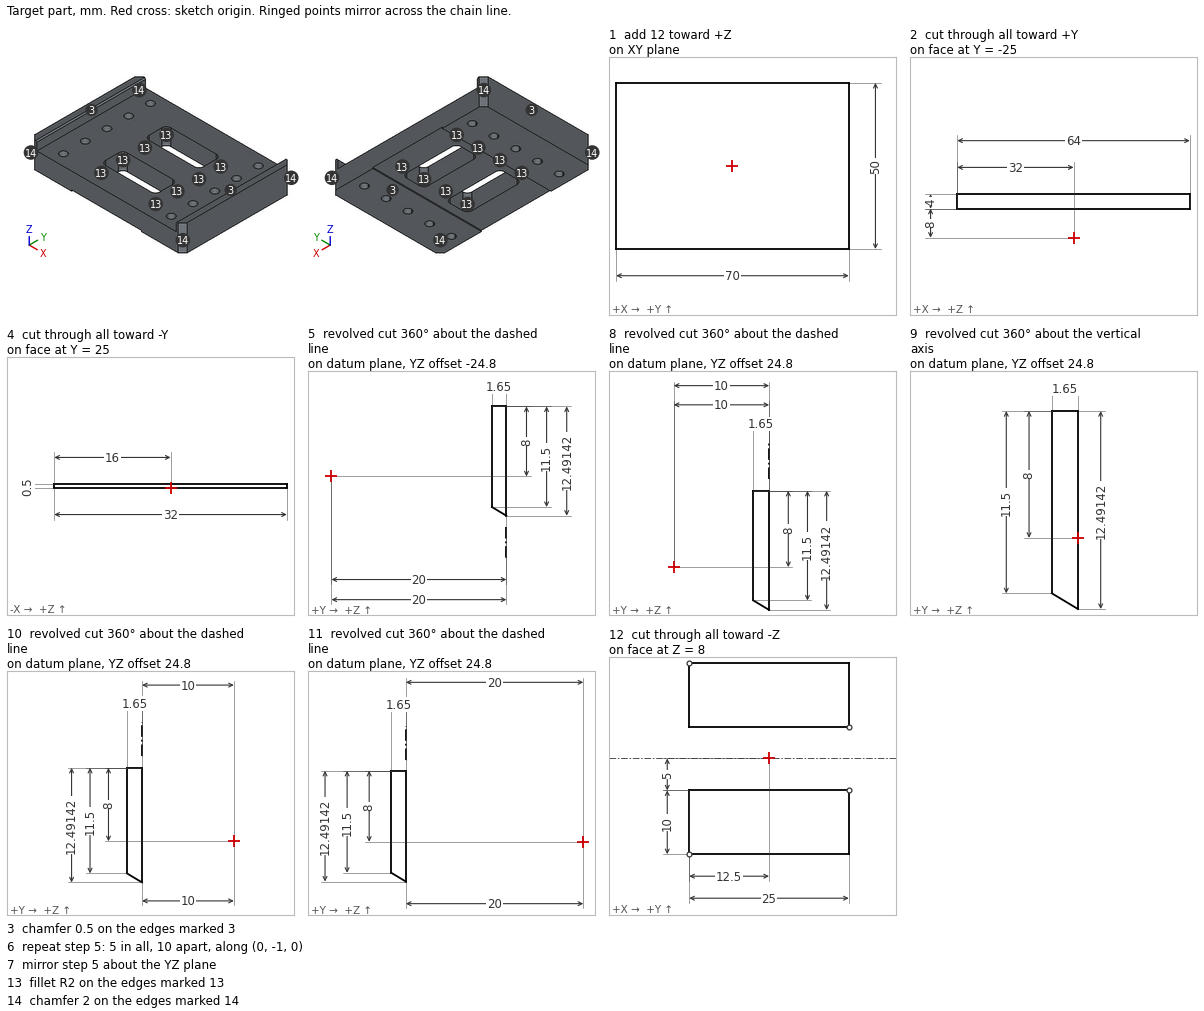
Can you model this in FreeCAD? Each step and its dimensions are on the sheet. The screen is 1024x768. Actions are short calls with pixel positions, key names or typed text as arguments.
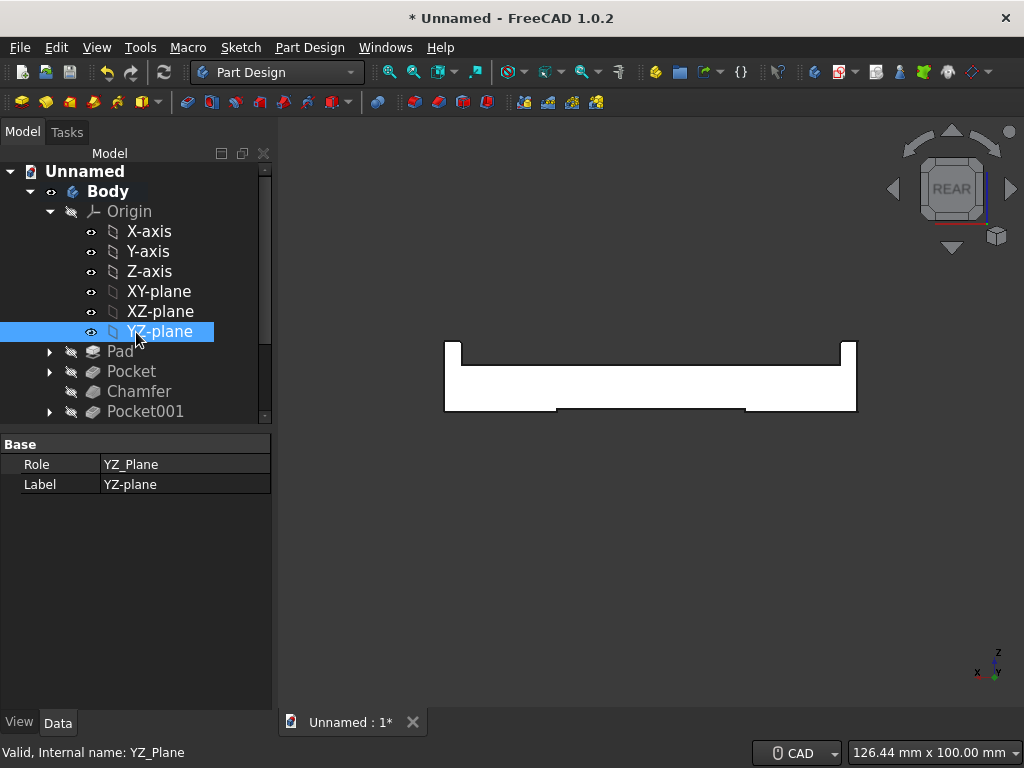
click(972, 72)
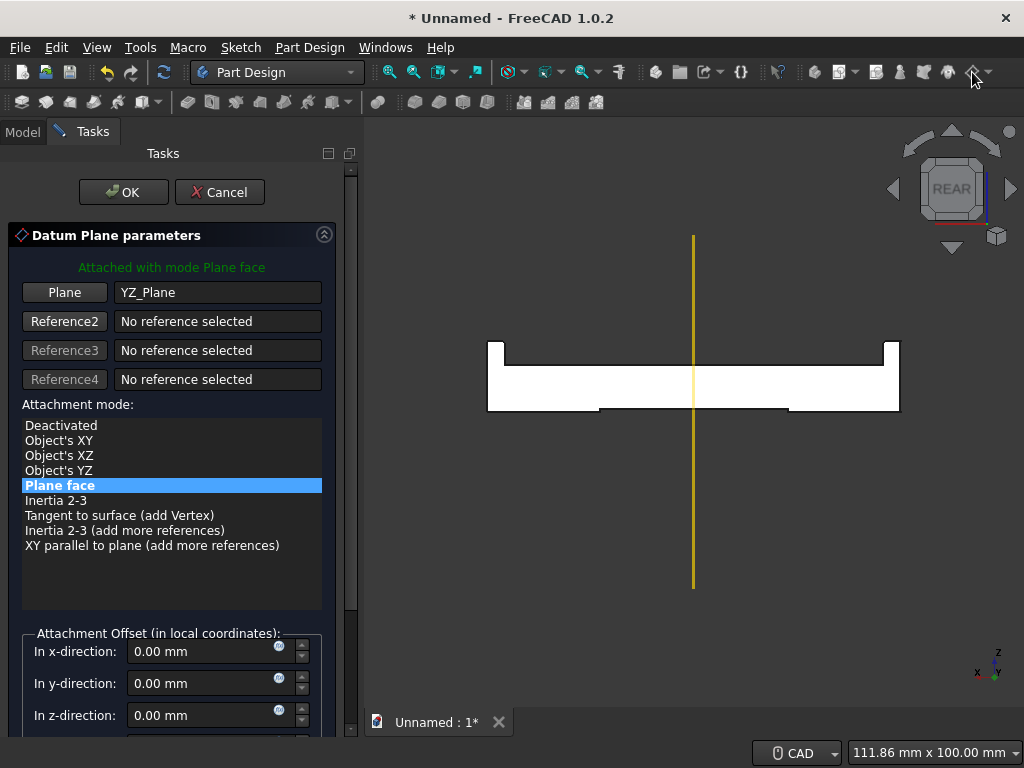
triple_click(210, 715)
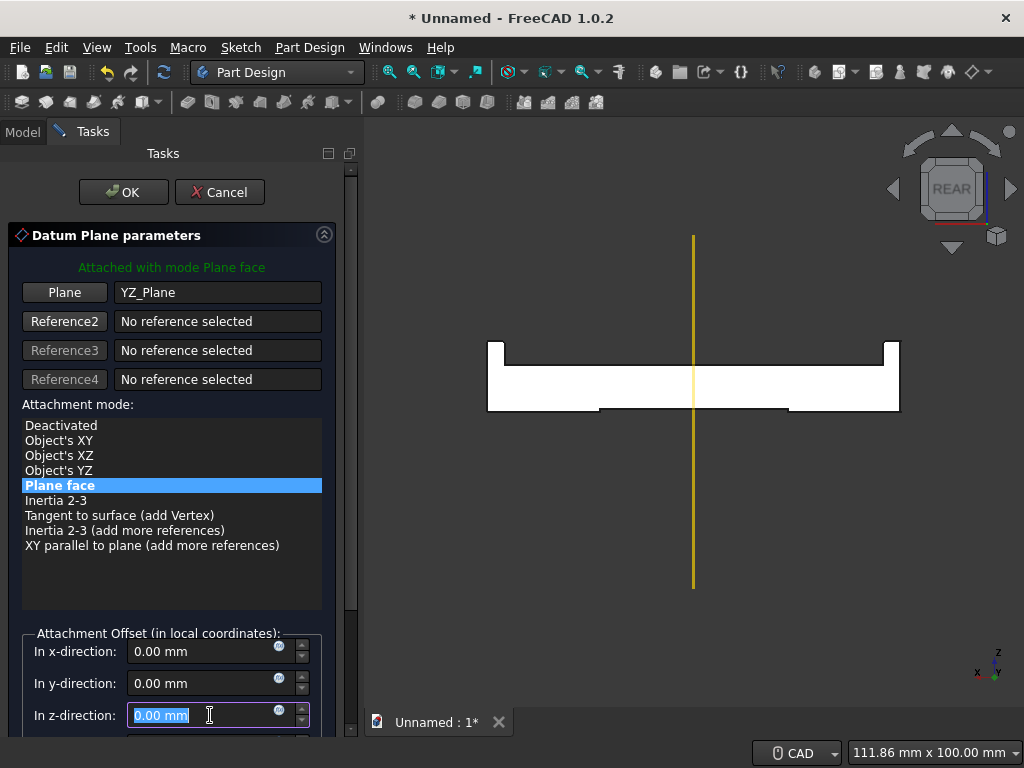
text(24.8)
key(Tab)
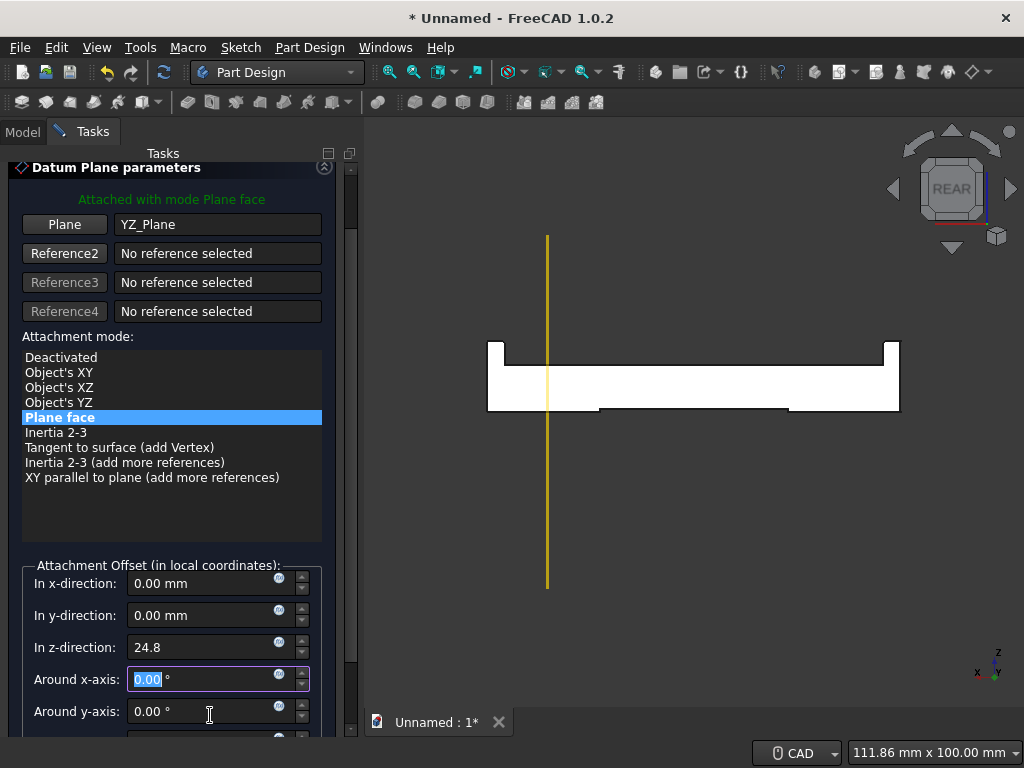
scroll(351, 450, up, 2)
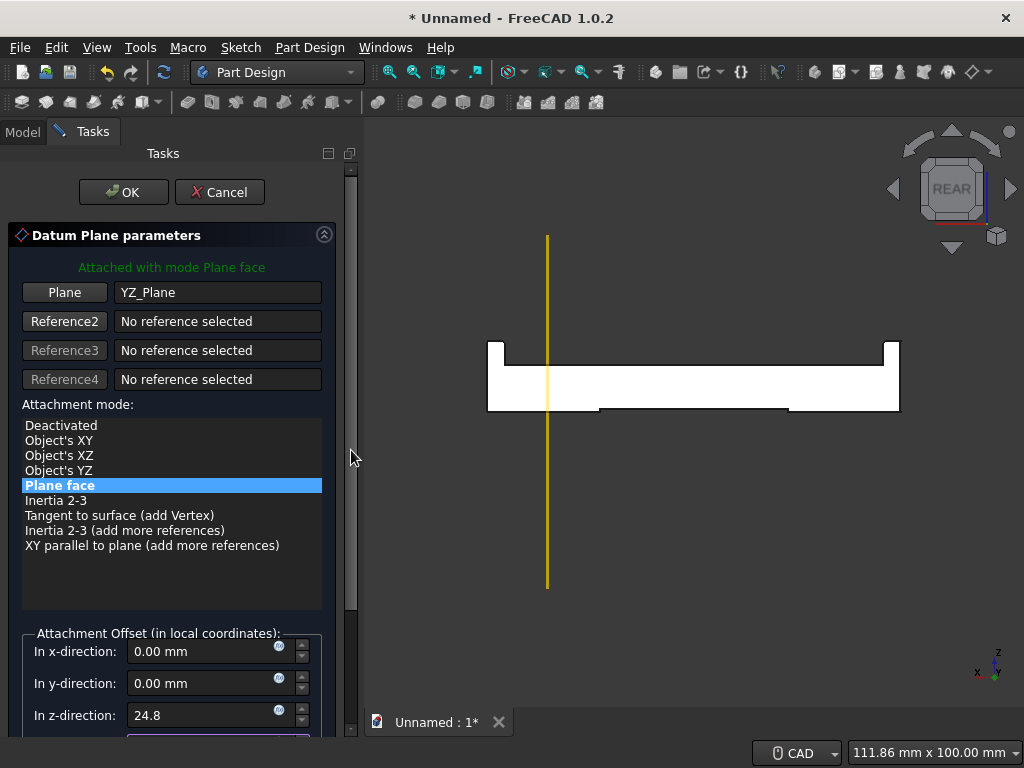
click(124, 192)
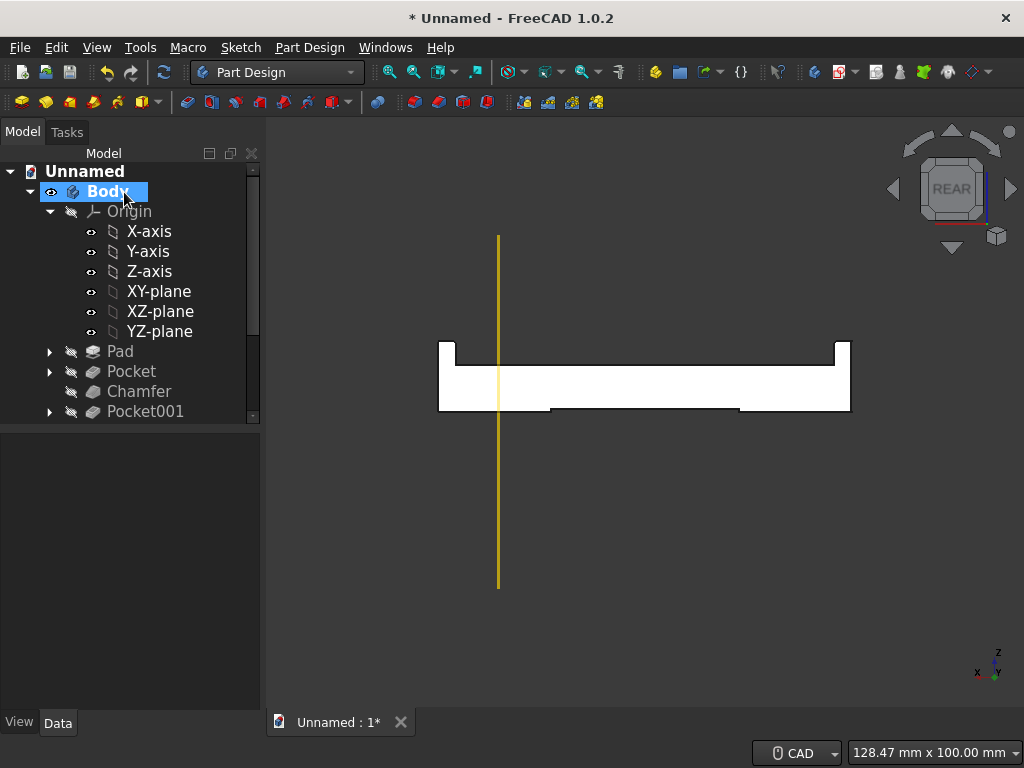
scroll(100, 287, down, 3)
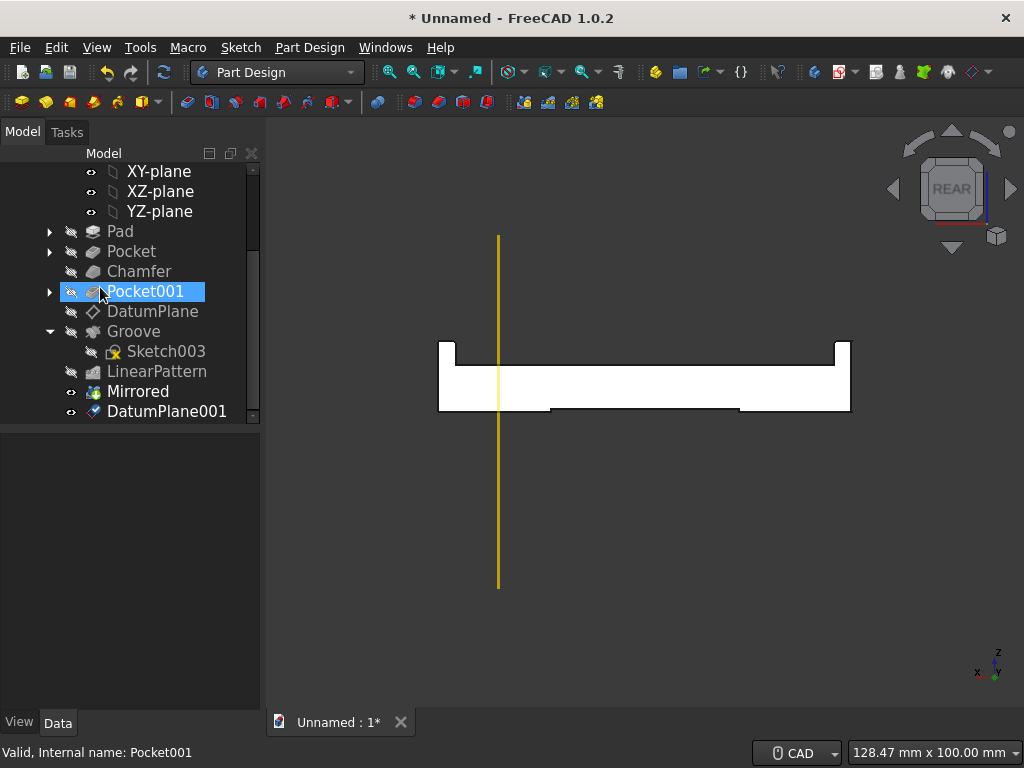
click(116, 412)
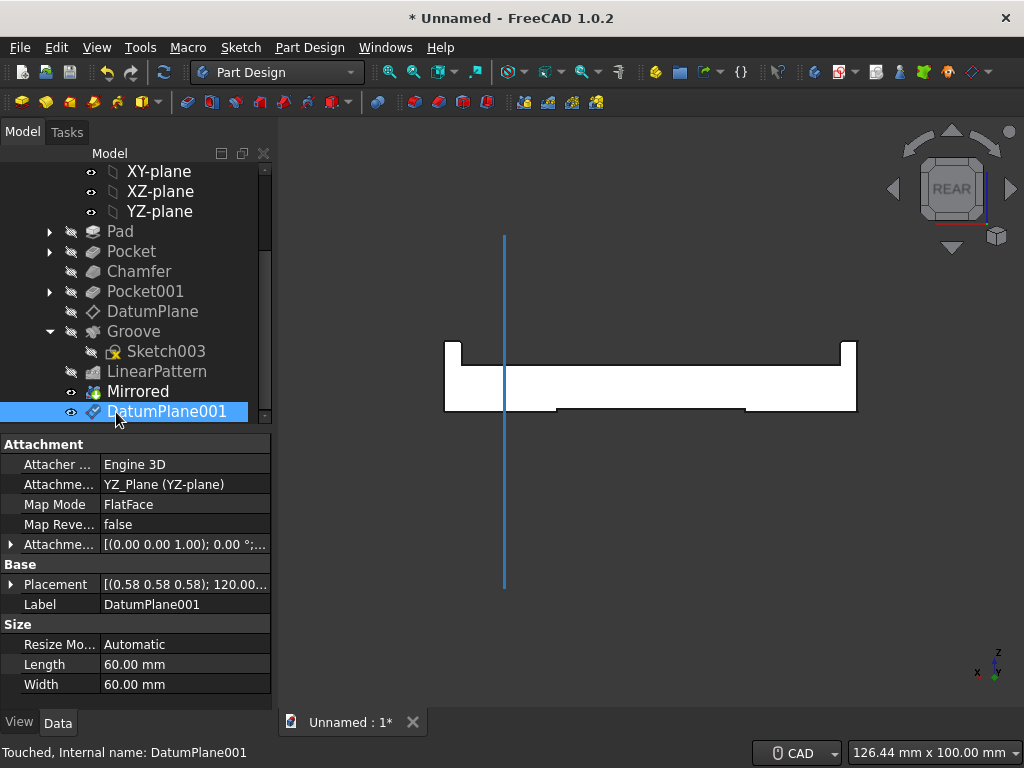
click(840, 72)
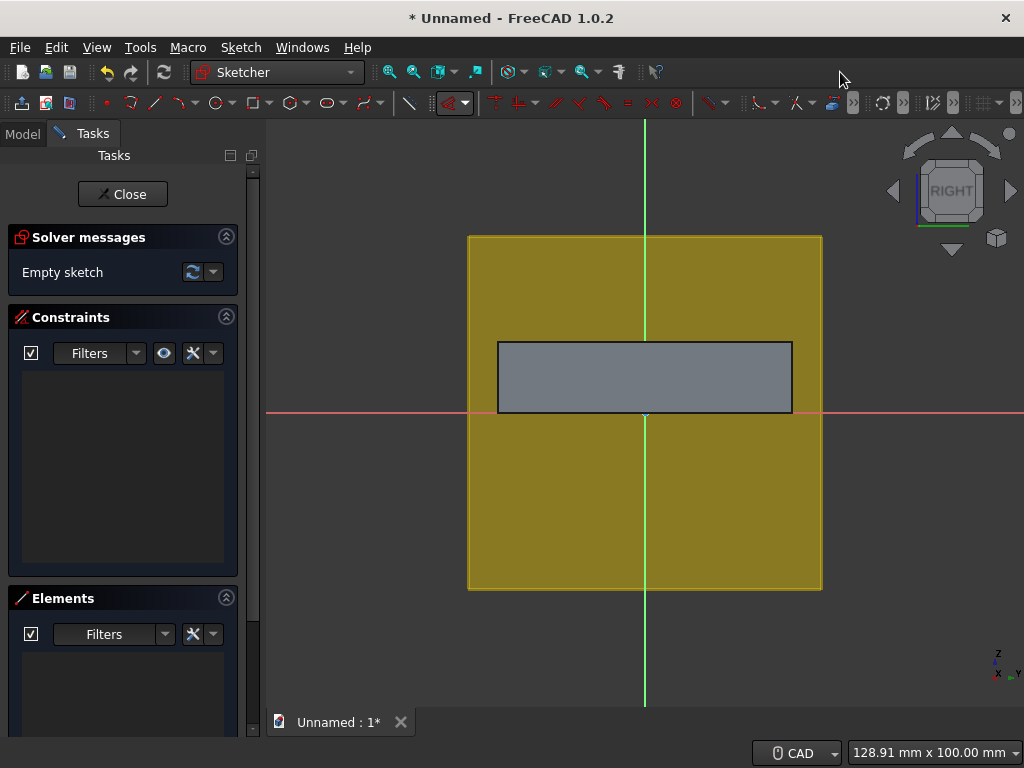
click(70, 104)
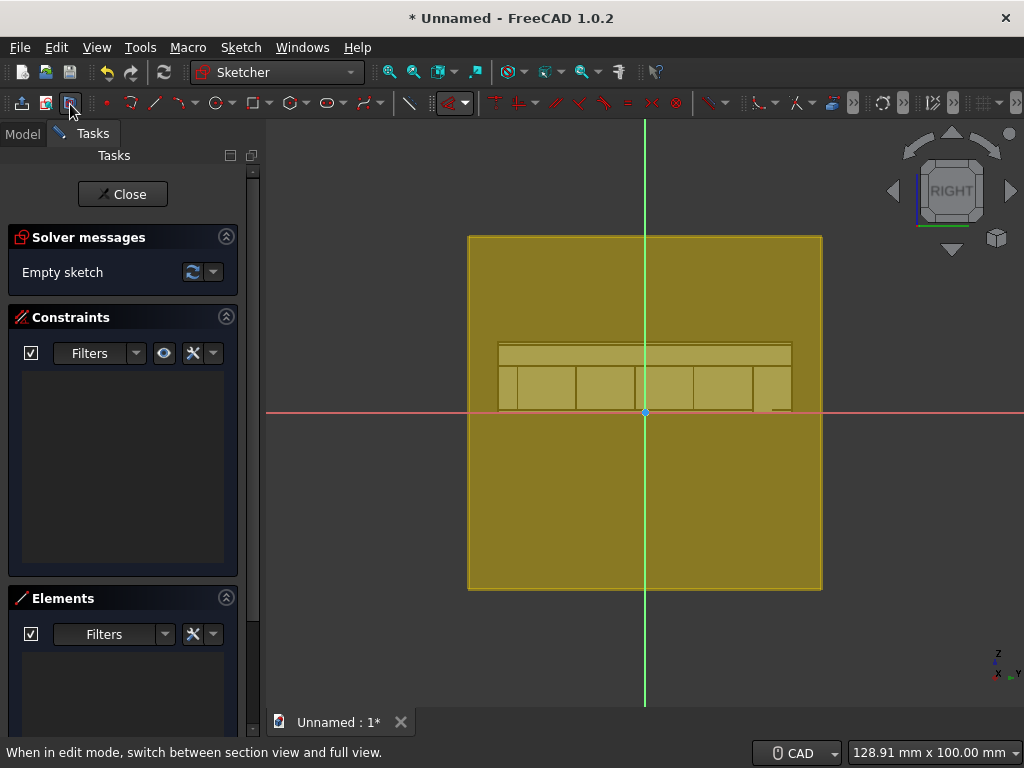
scroll(717, 377, up, 6)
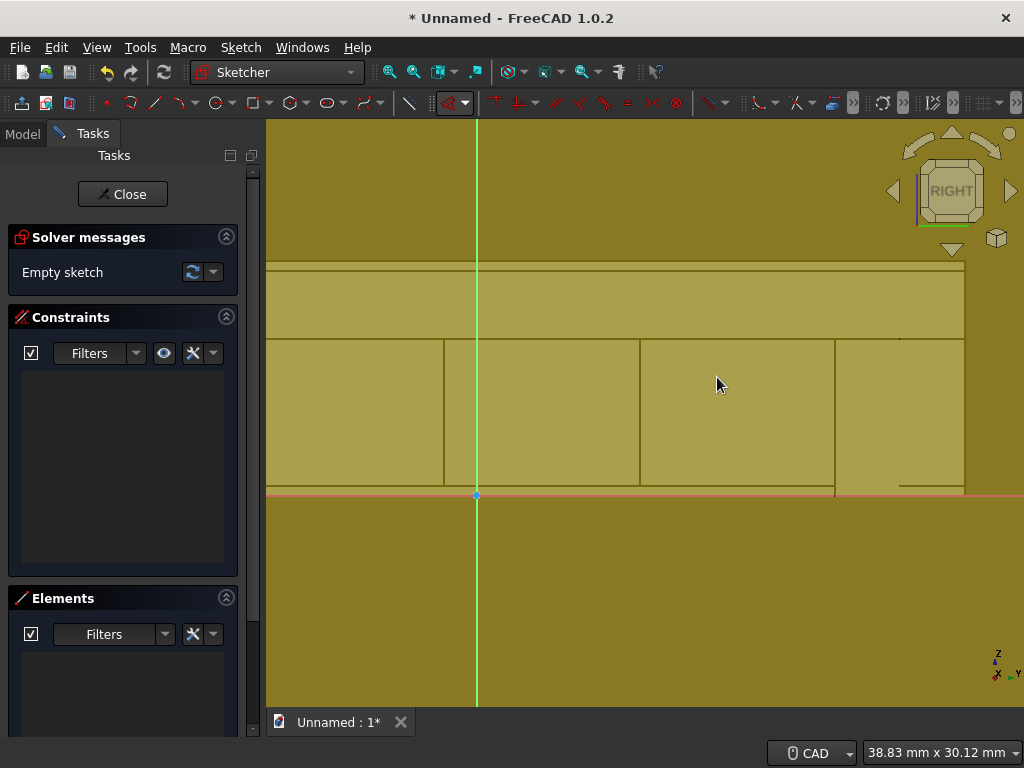
key(g)
key(m)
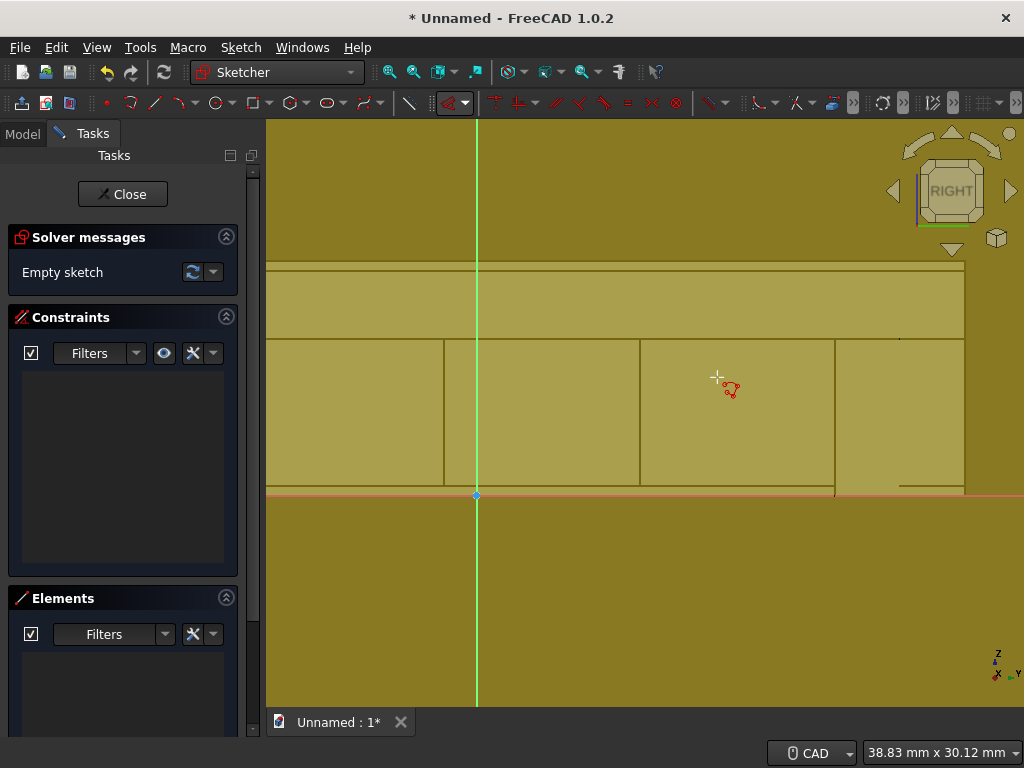
click(640, 564)
click(640, 339)
click(672, 339)
click(672, 583)
click(640, 565)